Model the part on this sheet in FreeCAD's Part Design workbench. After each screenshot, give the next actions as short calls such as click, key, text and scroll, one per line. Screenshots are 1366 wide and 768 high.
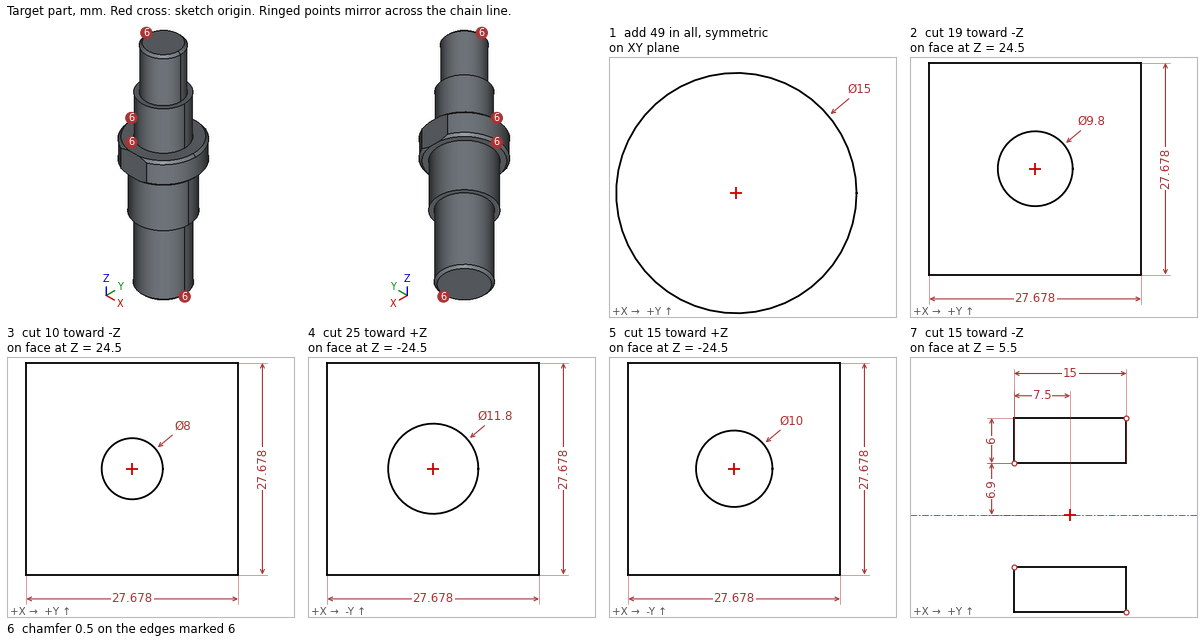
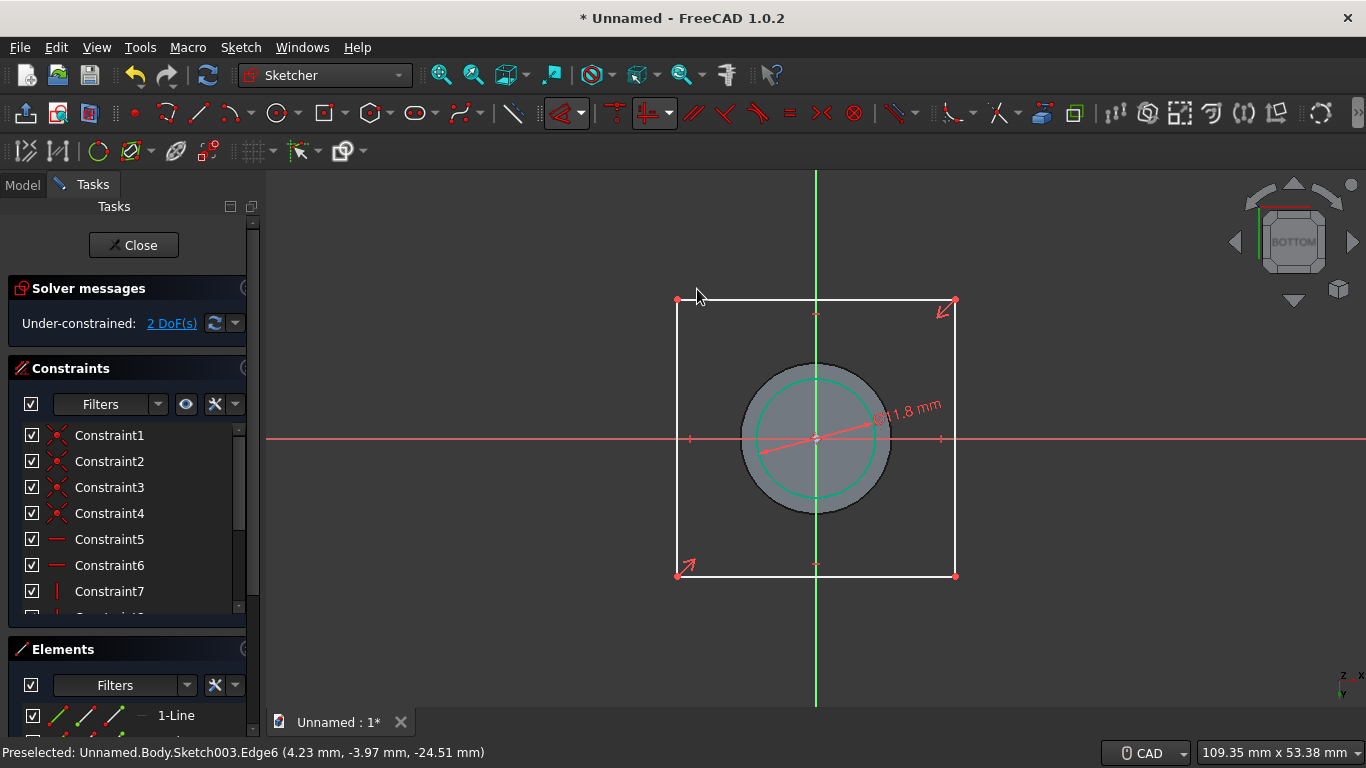
click(760, 577)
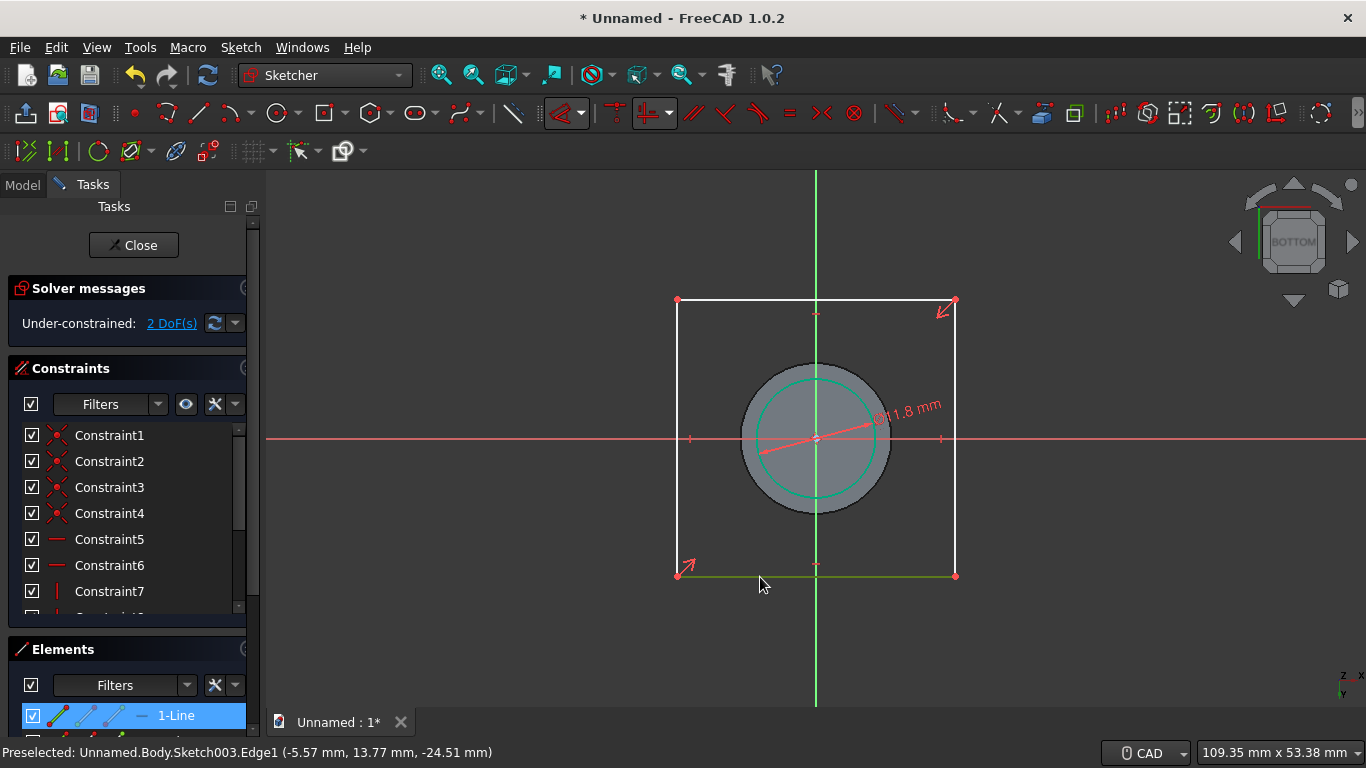
key(l)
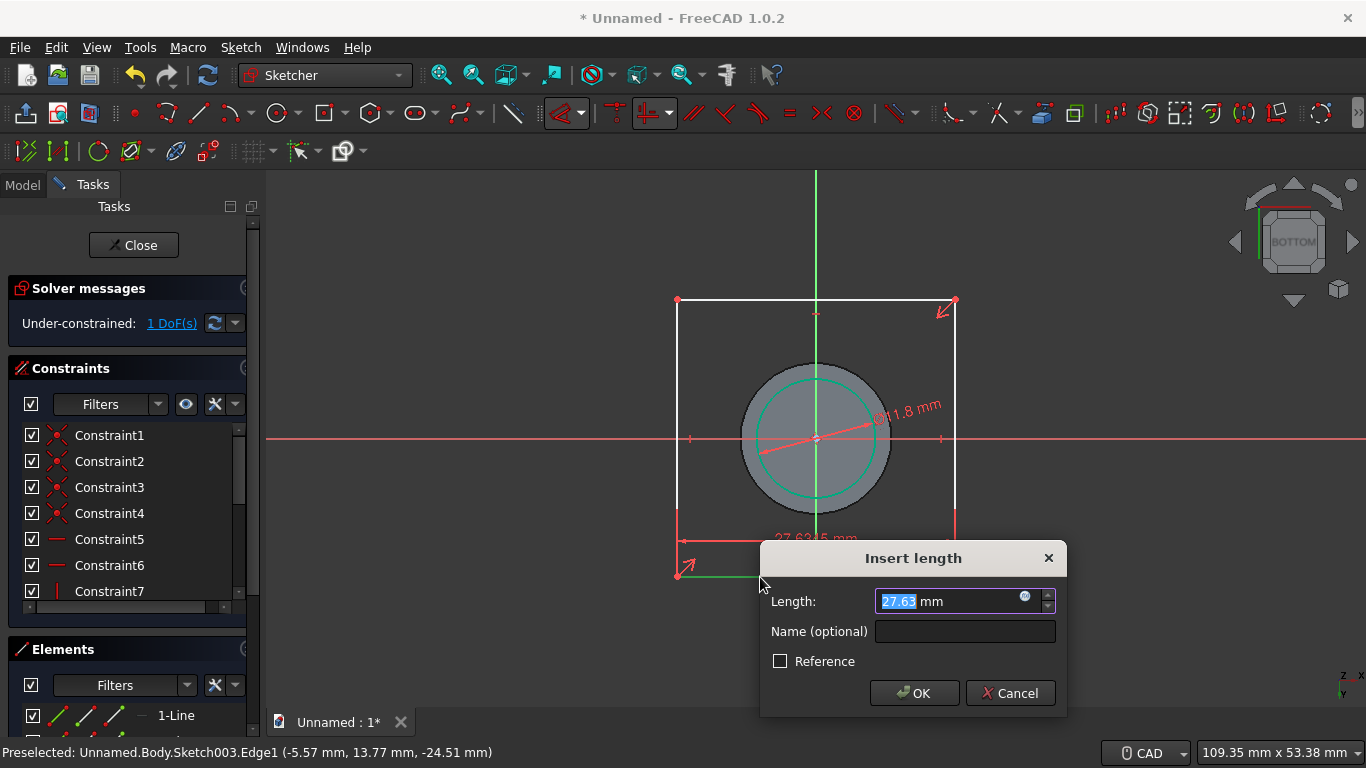
text(27.678)
key(Return)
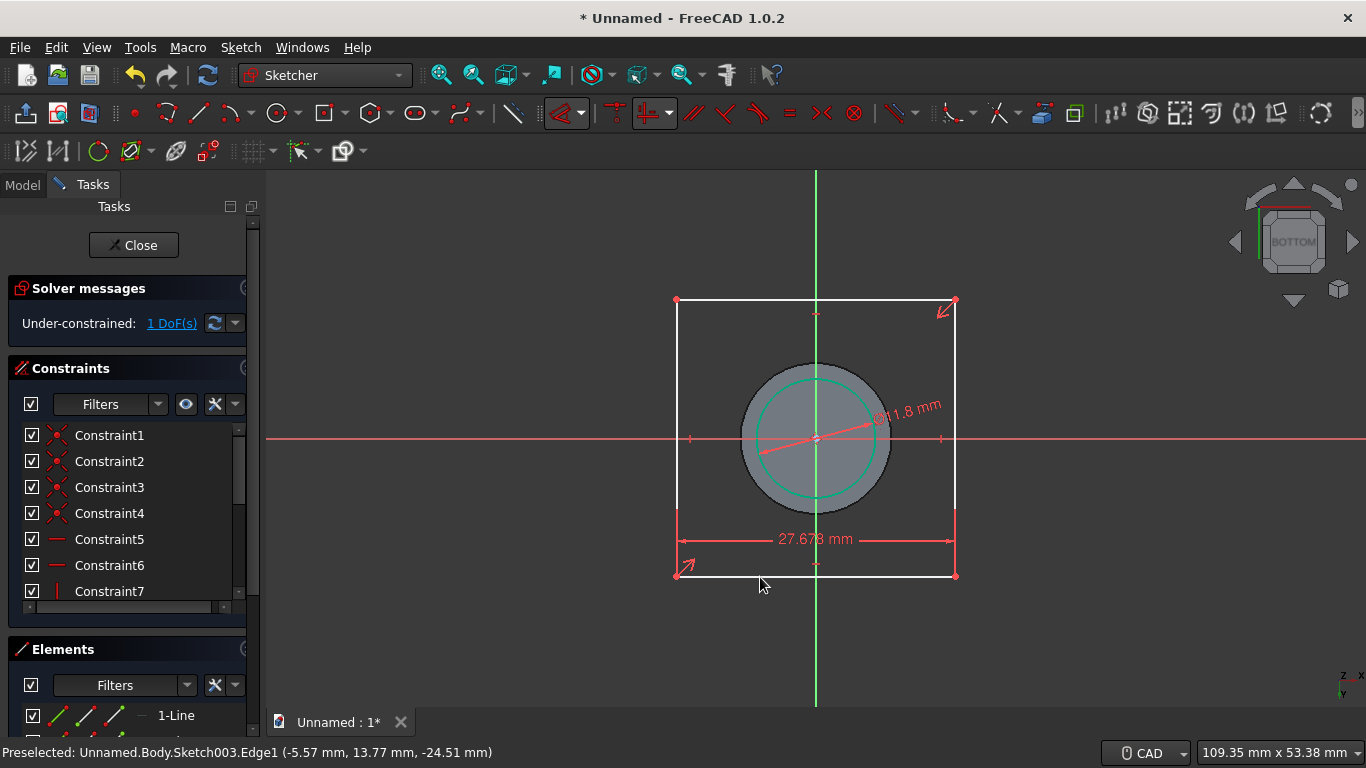
click(955, 494)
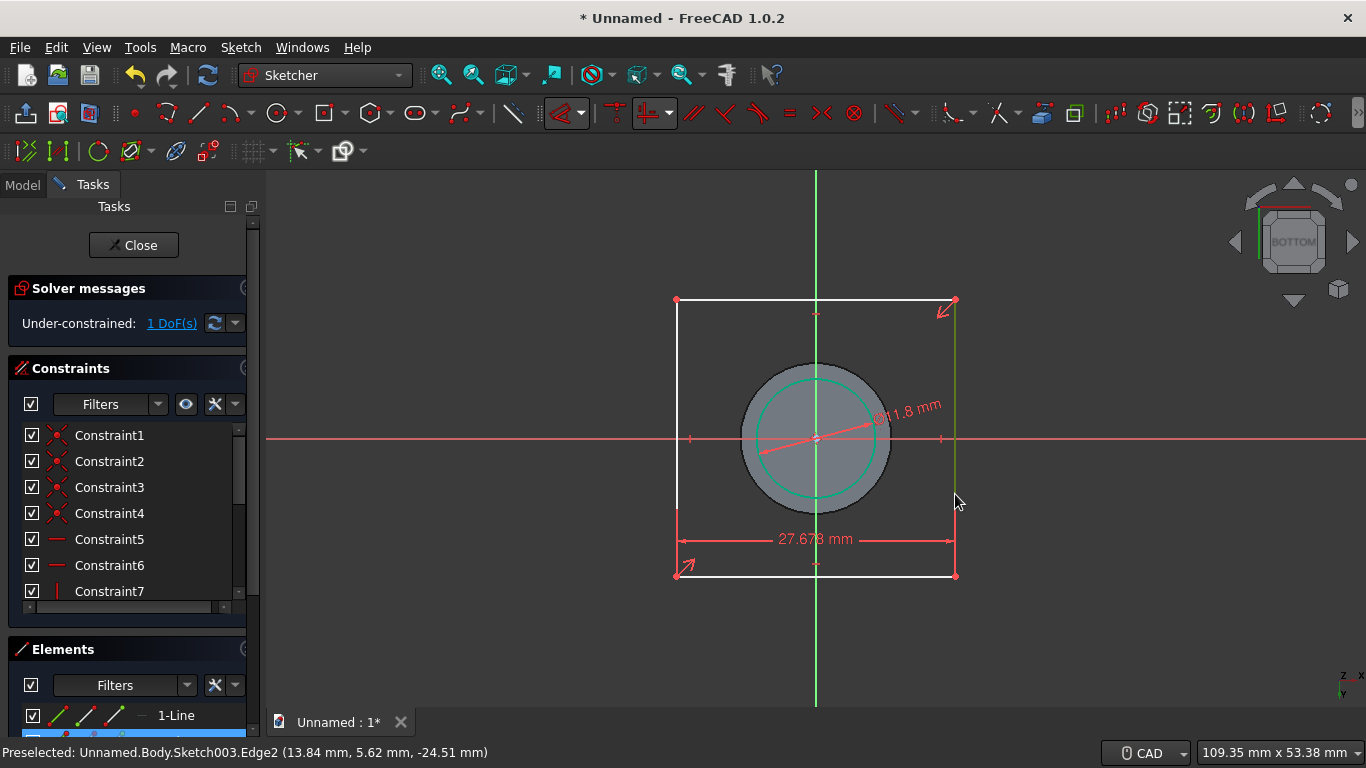
key(i)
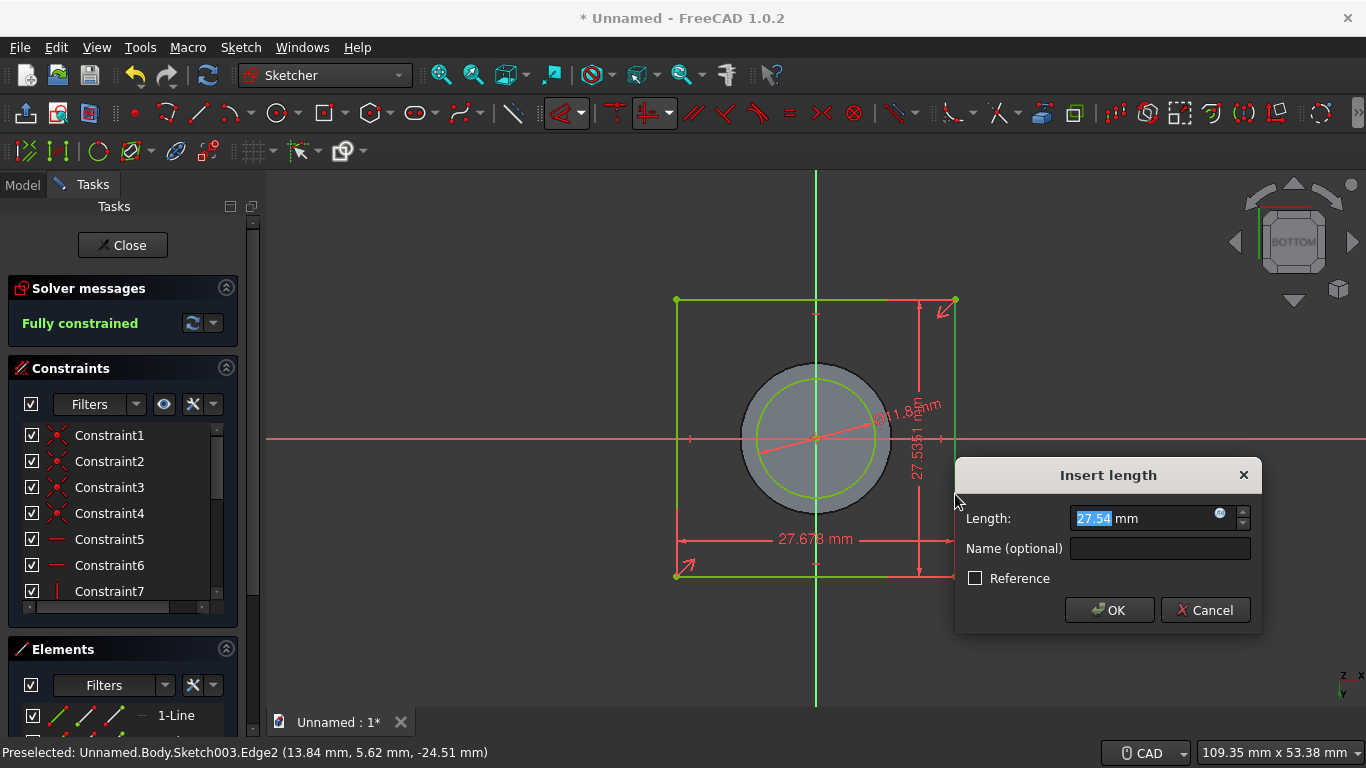
text(27.678)
key(Return)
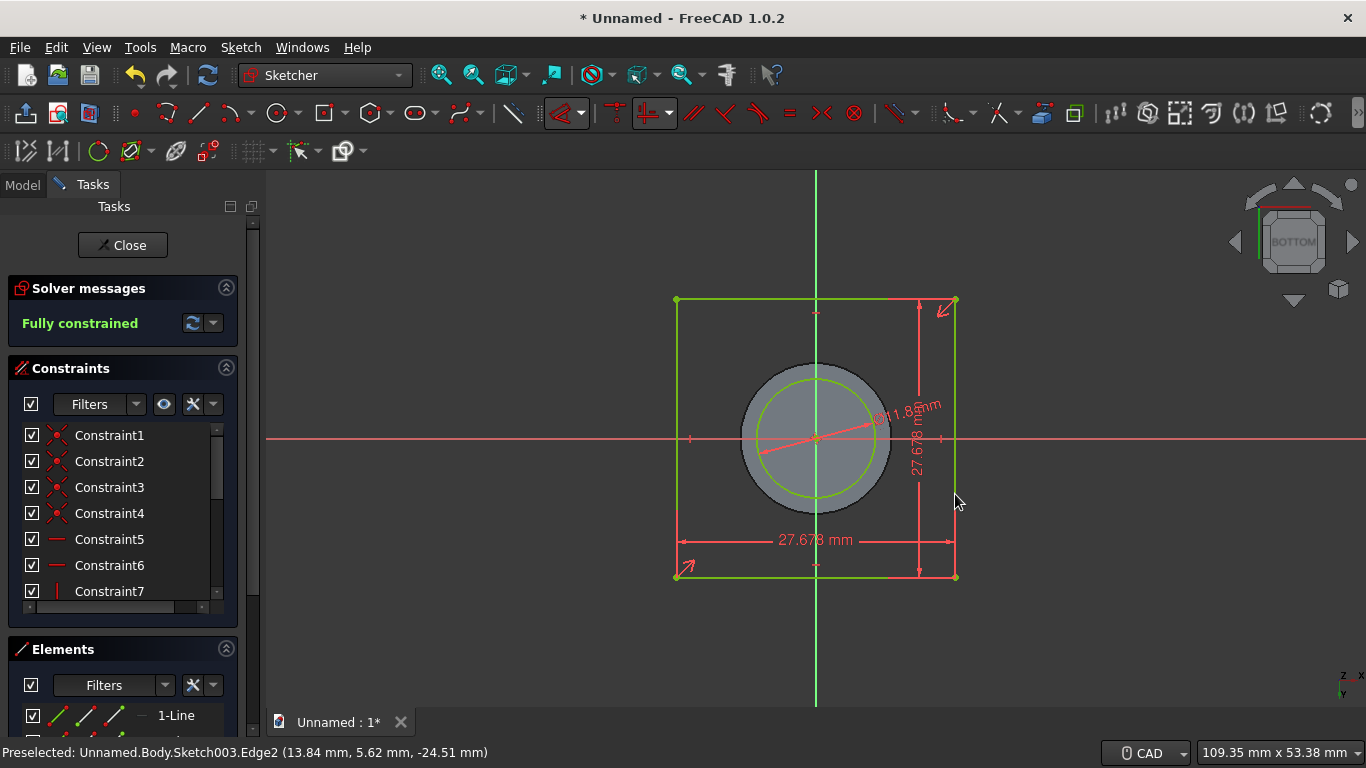
click(123, 245)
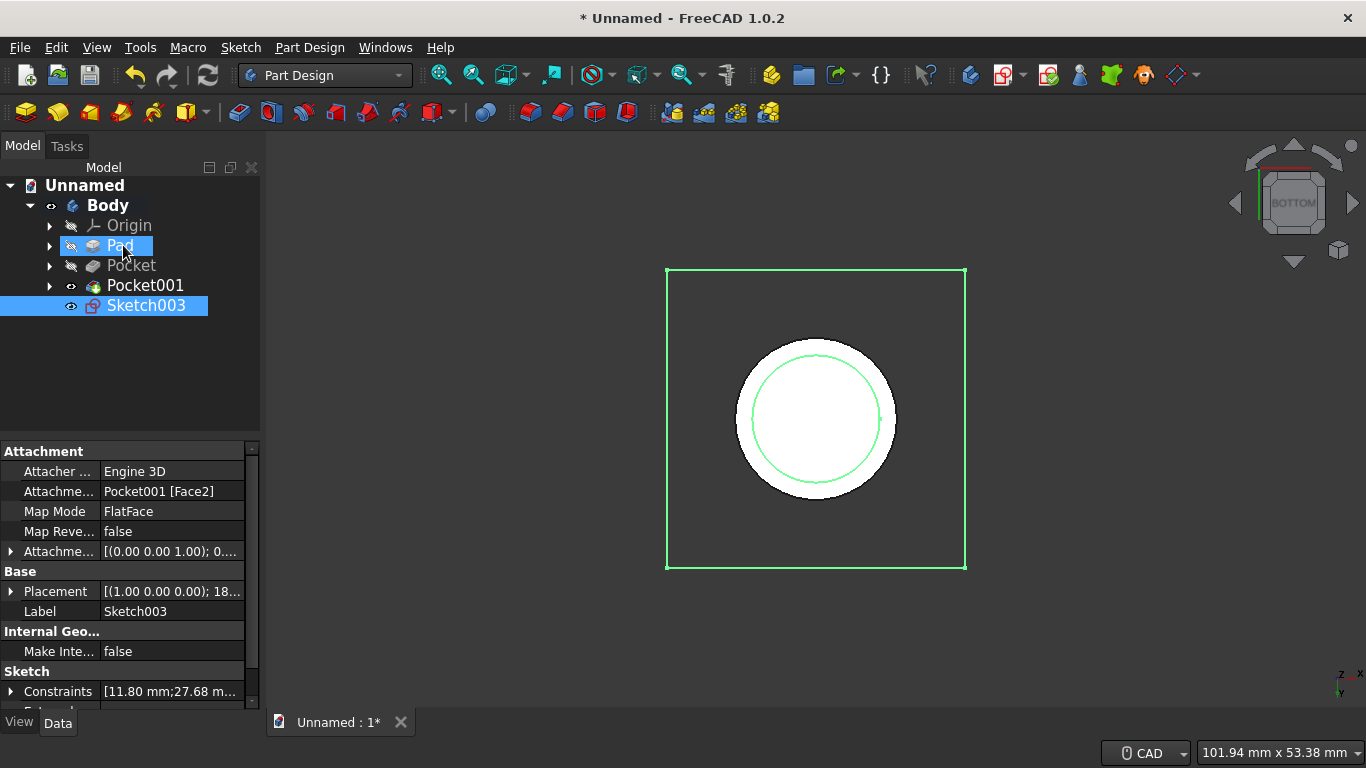
click(240, 112)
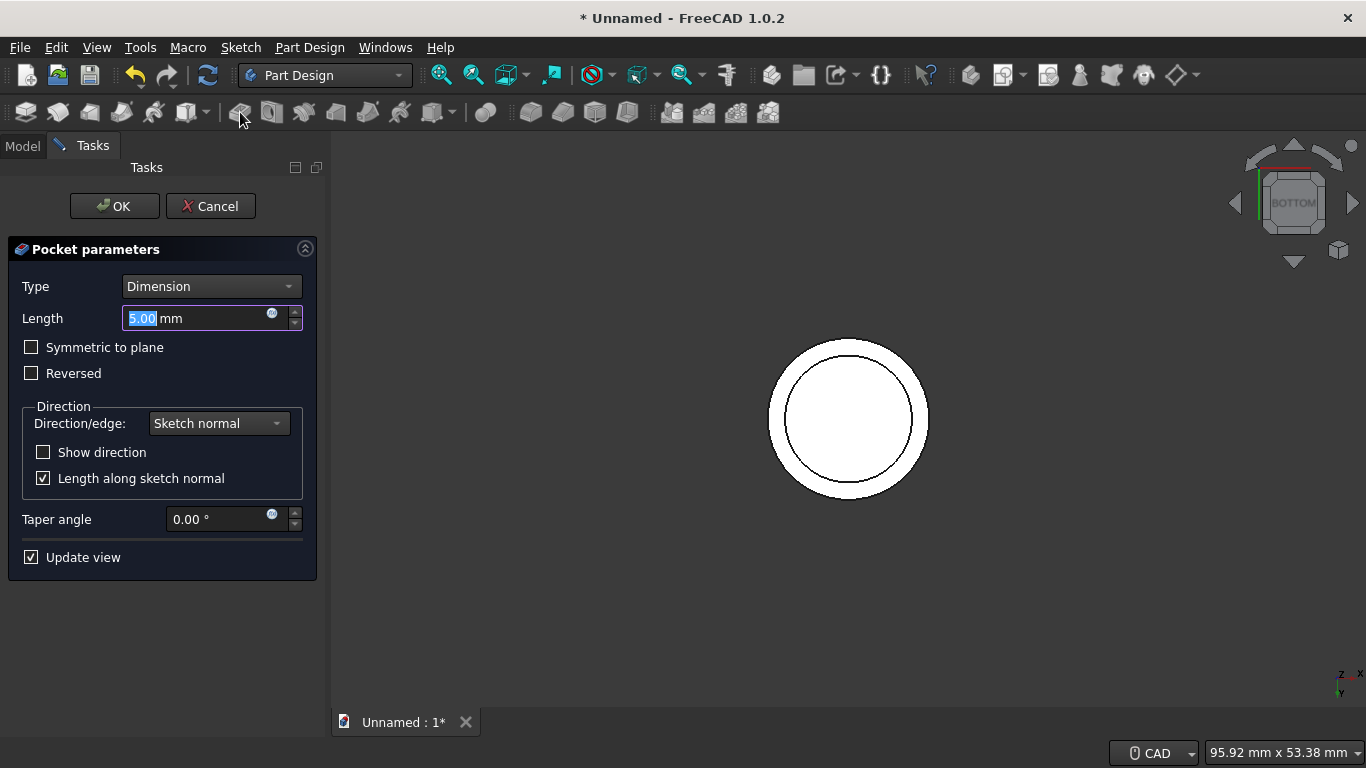
text(25)
key(Tab)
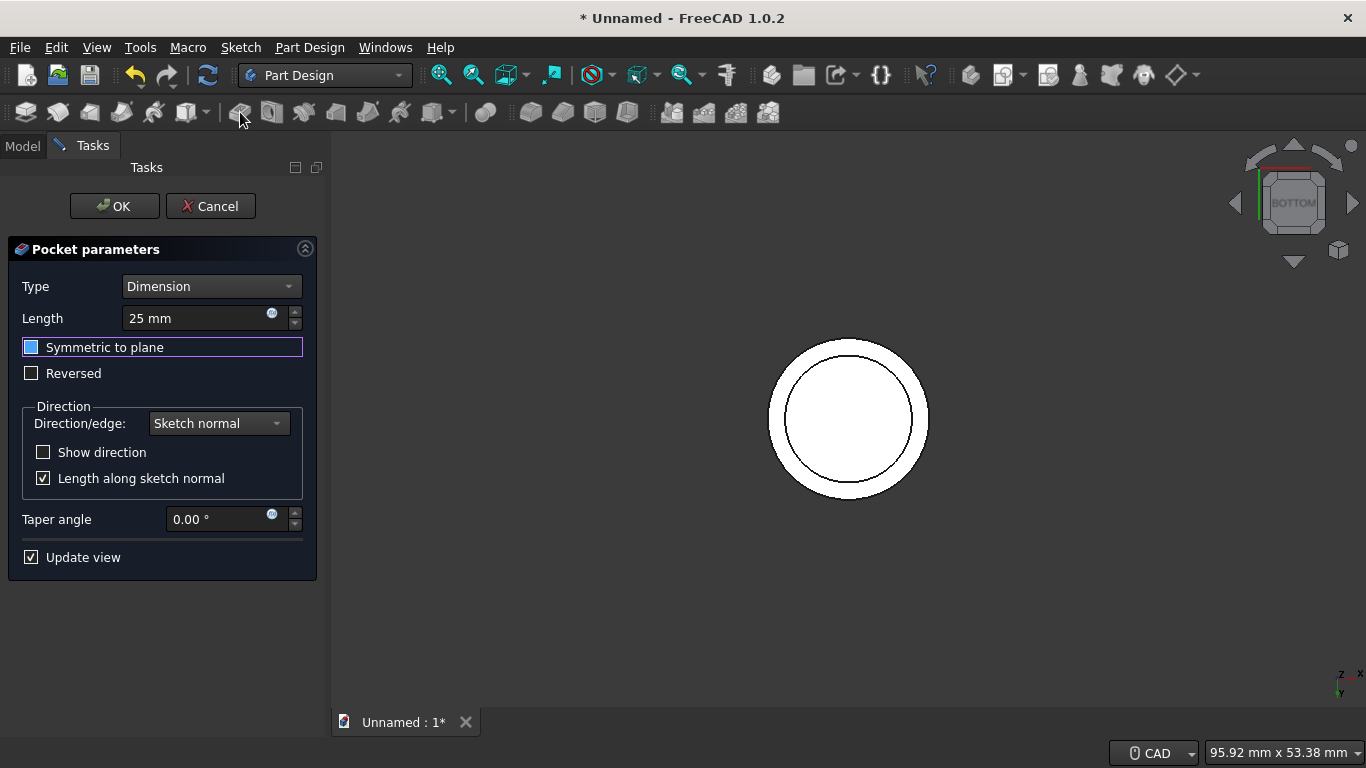
click(115, 206)